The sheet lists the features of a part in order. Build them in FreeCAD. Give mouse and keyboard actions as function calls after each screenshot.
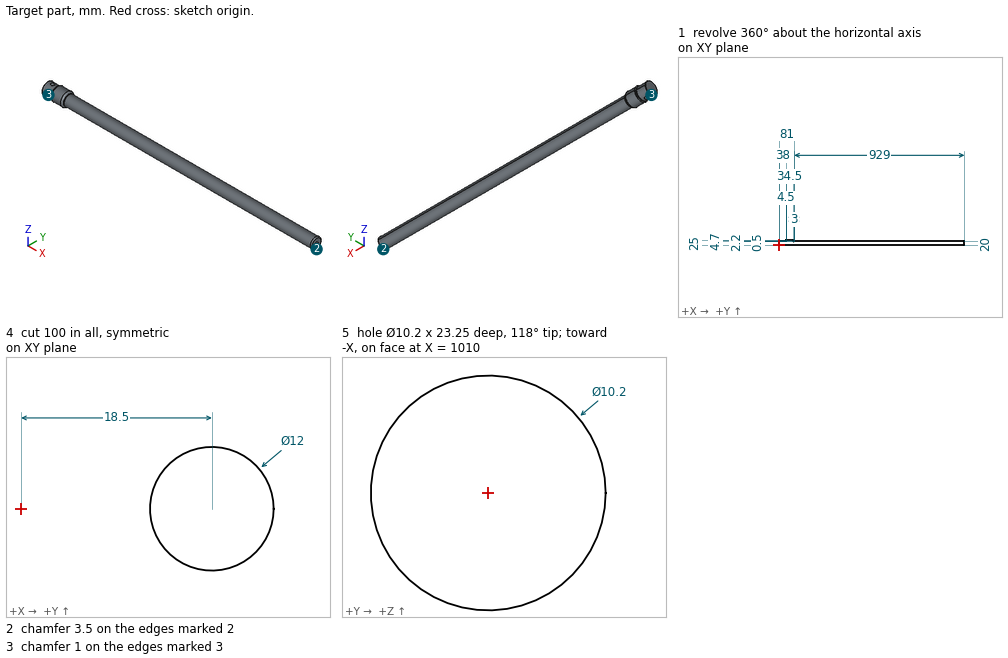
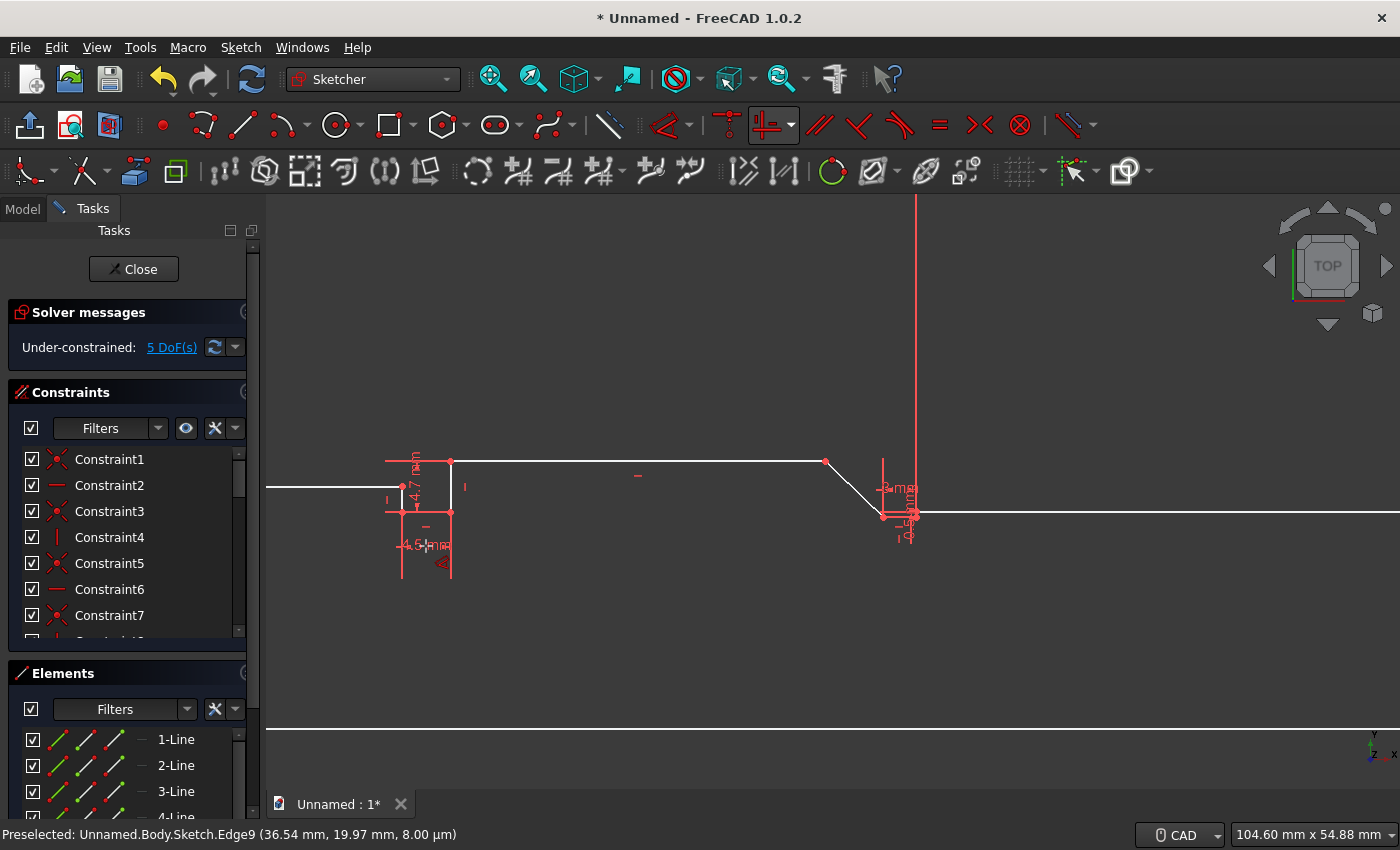
scroll(402, 502, up, 3)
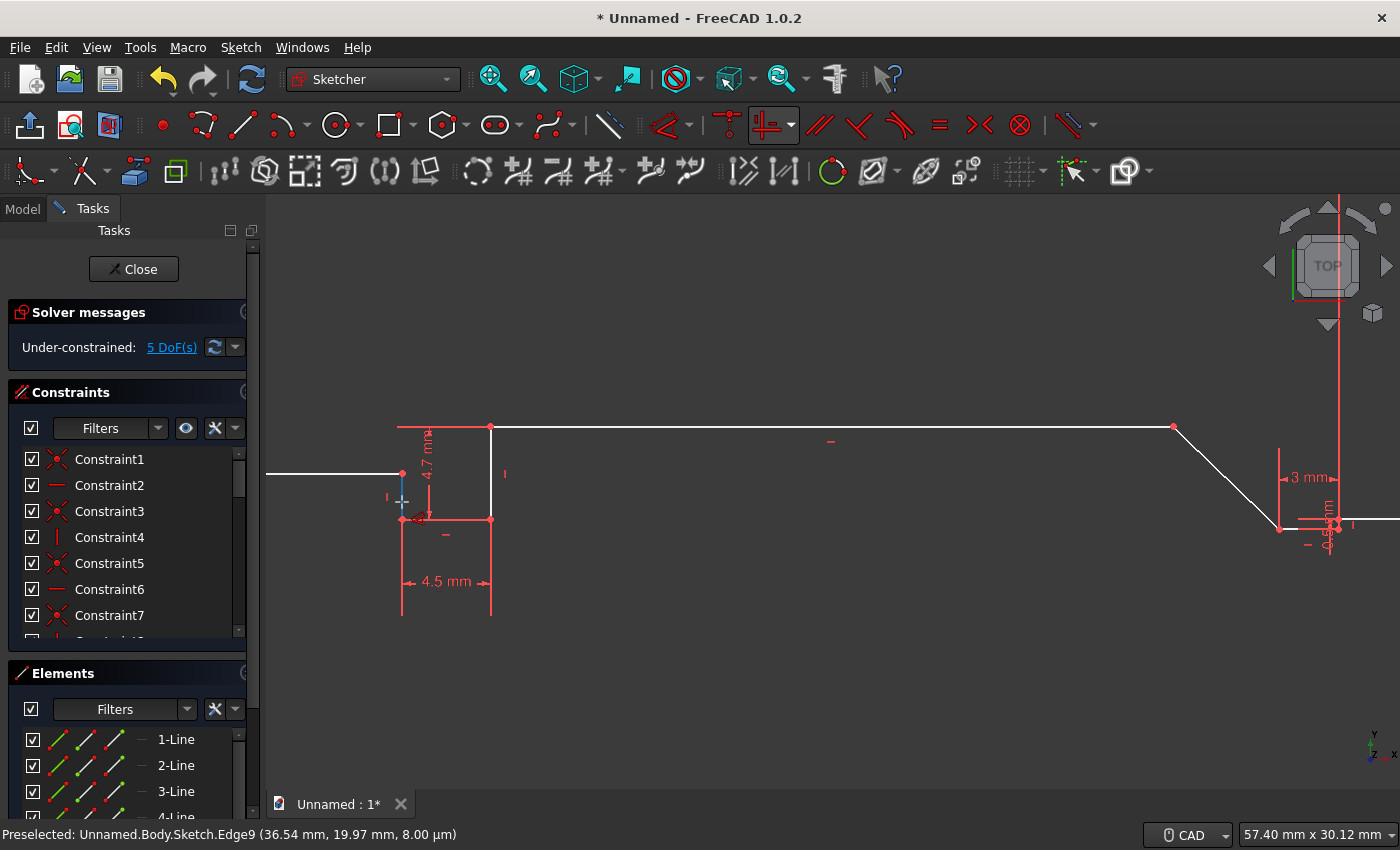
click(402, 501)
click(368, 497)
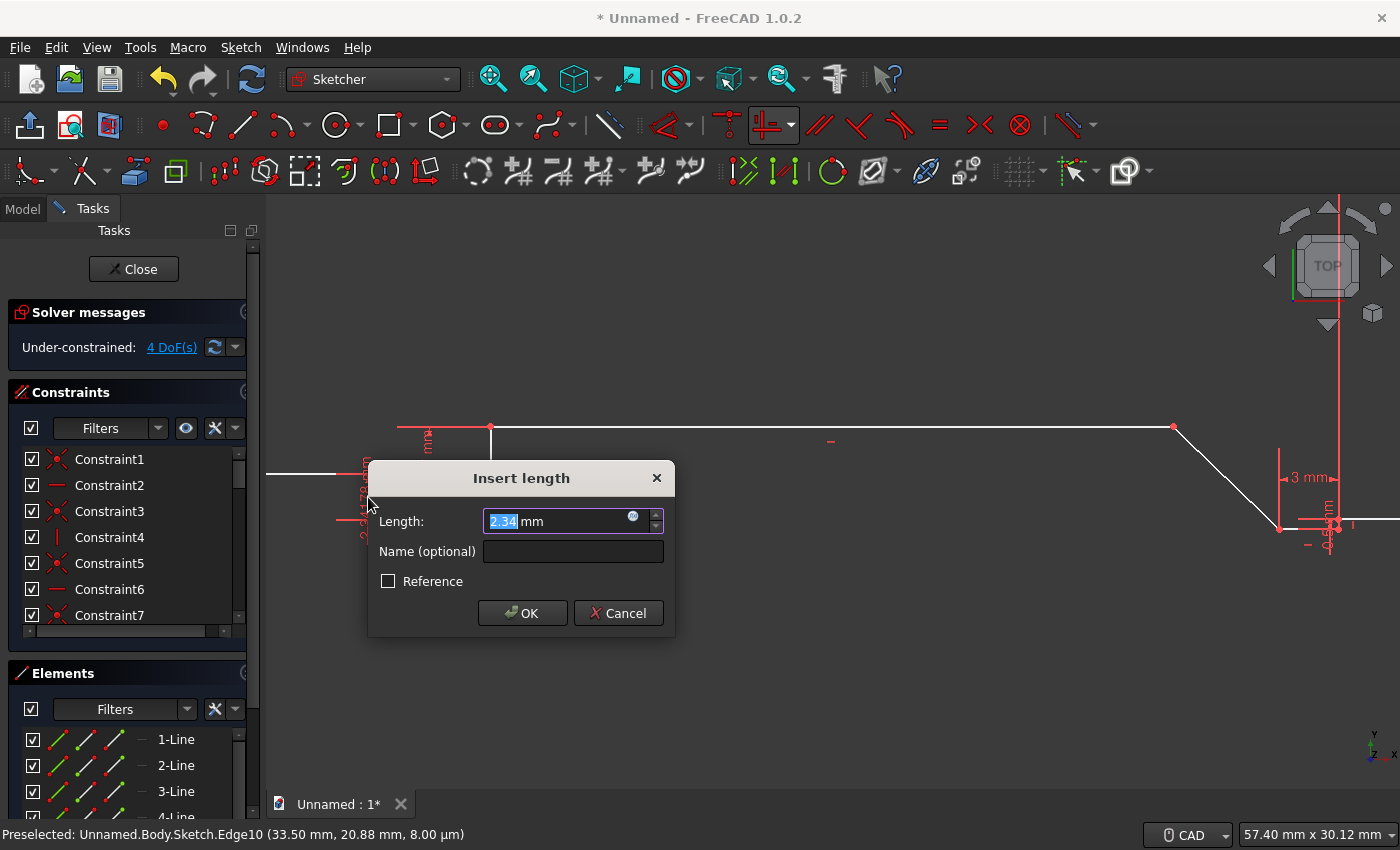
text(2.2)
key(Return)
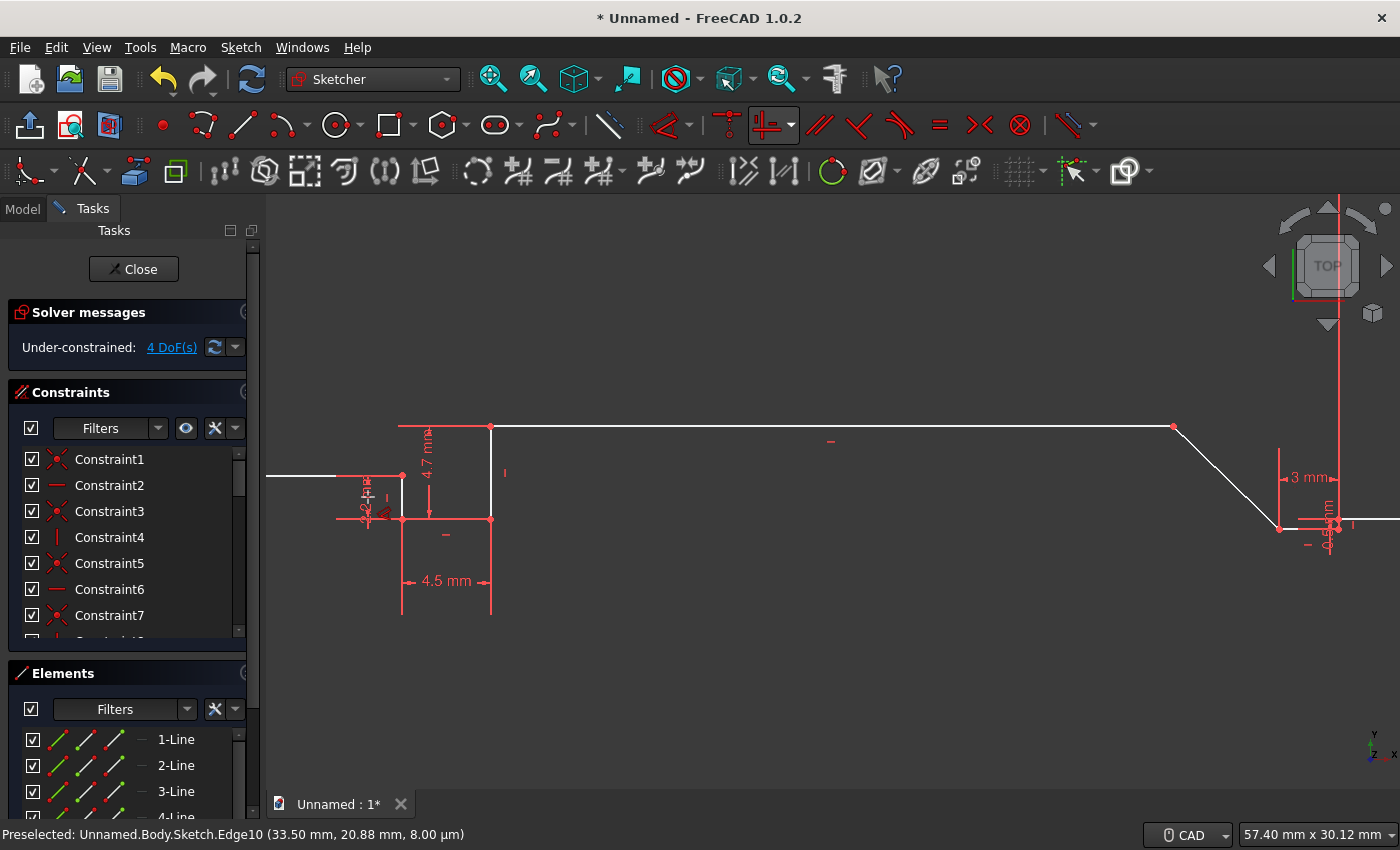
scroll(384, 484, down, 16)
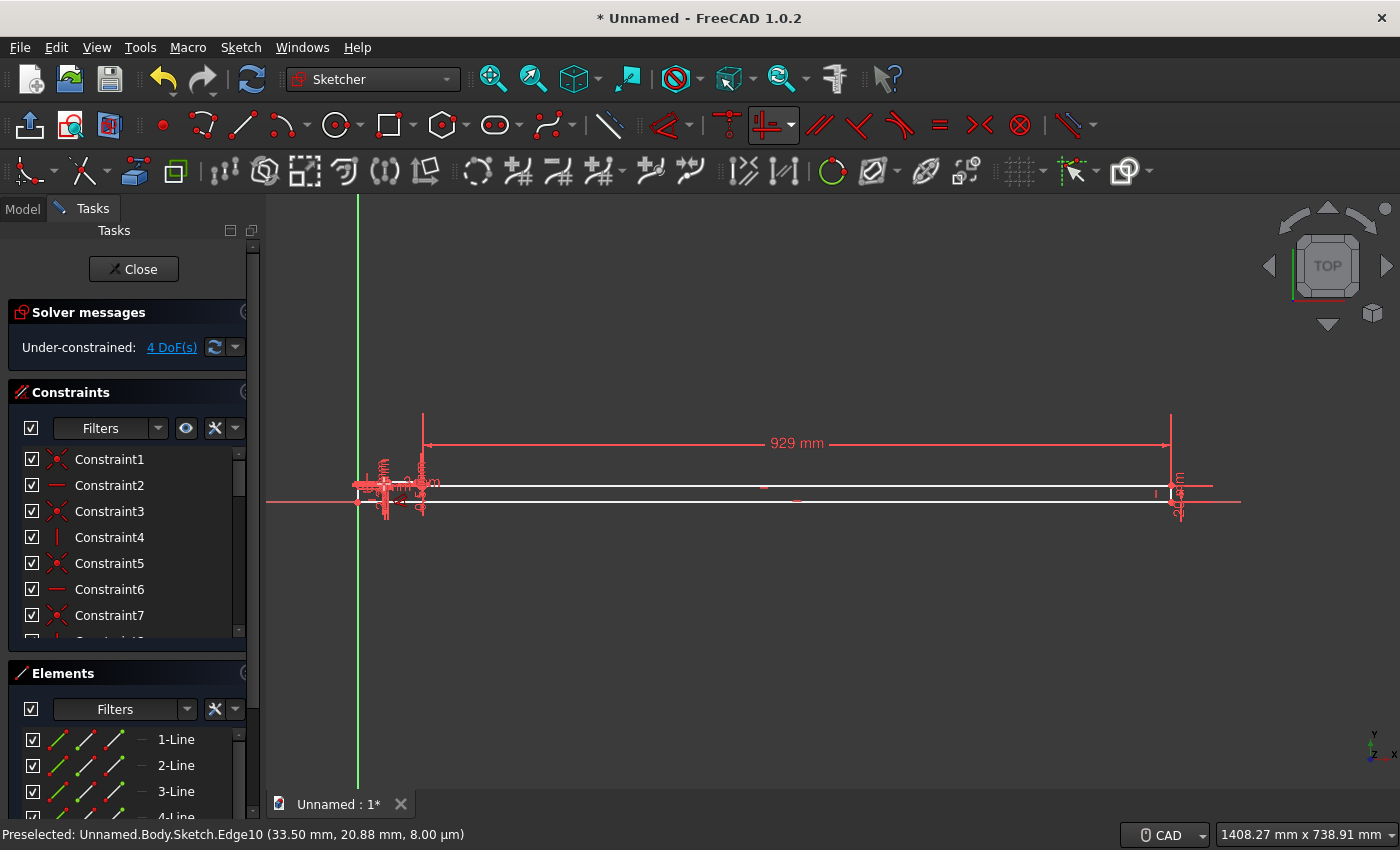
scroll(423, 486, up, 13)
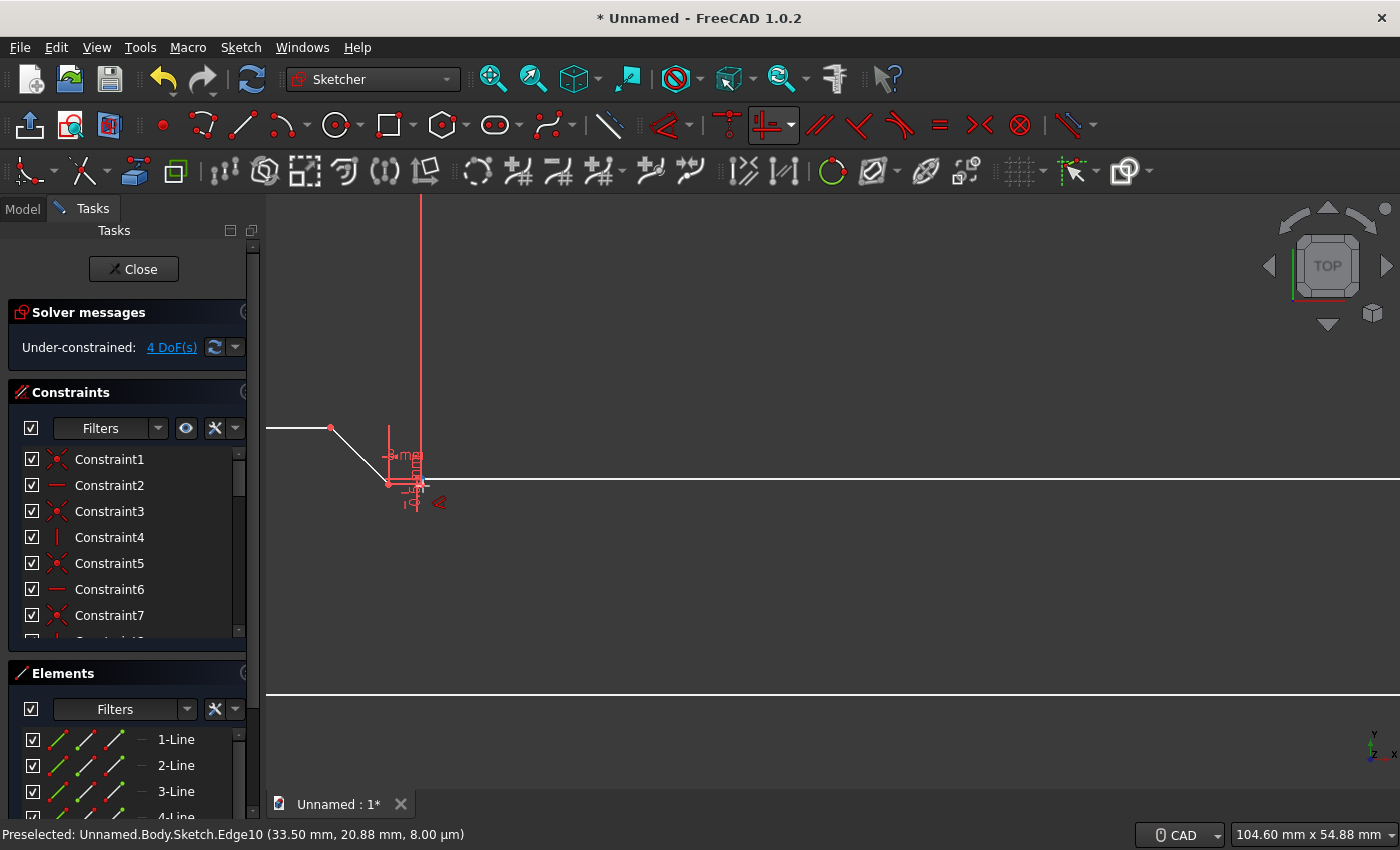
click(421, 479)
click(358, 729)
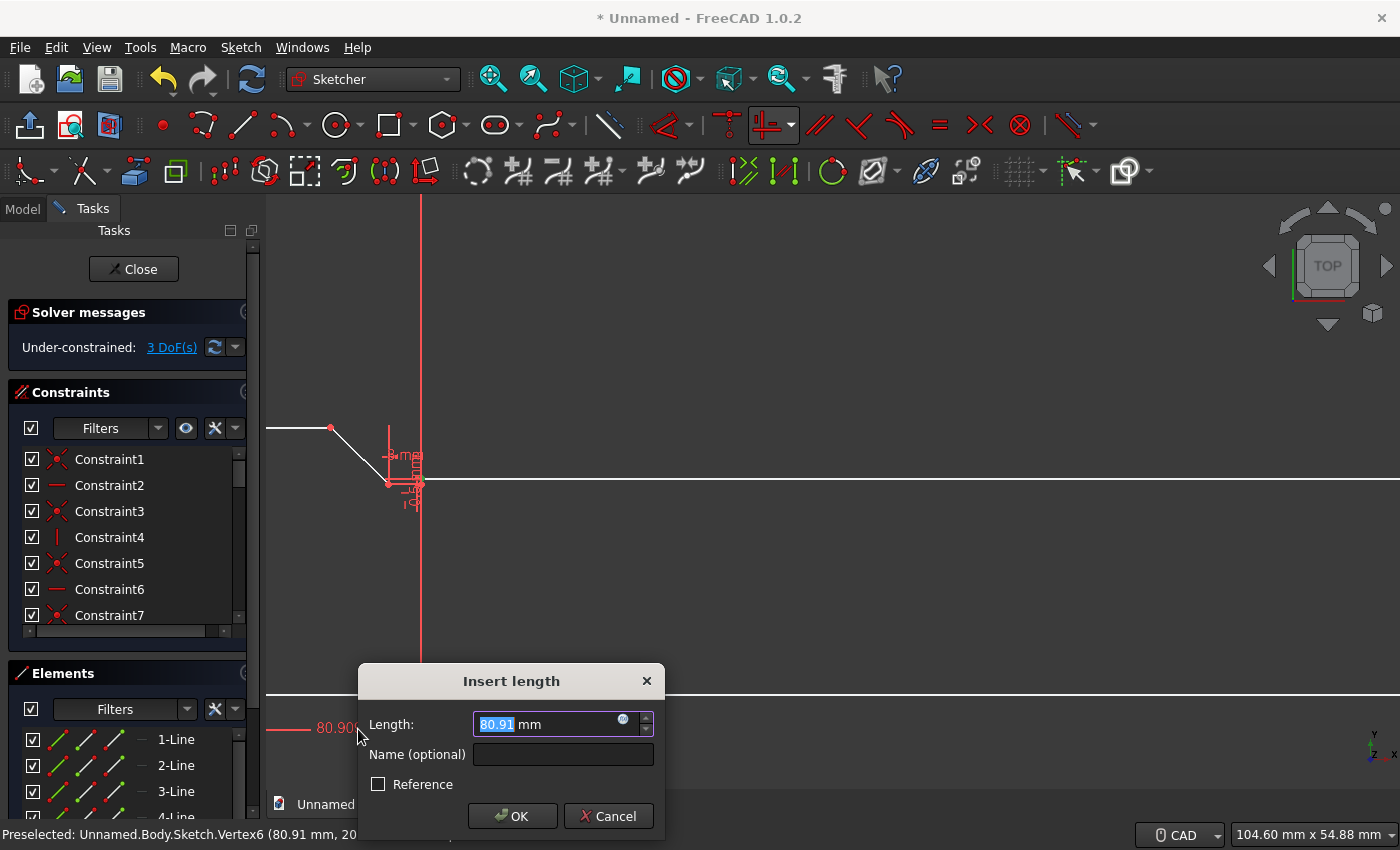
text(81)
key(Return)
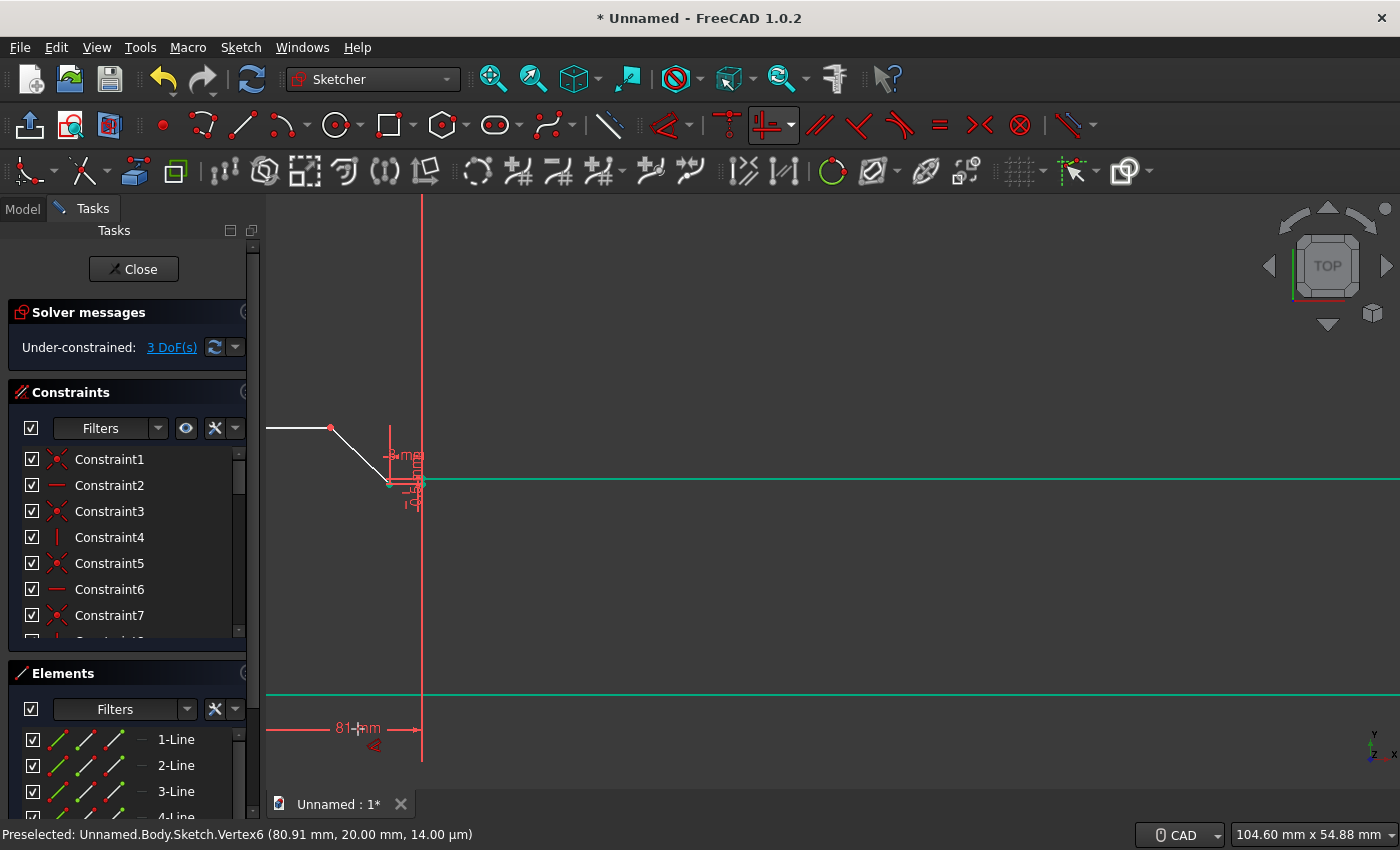
scroll(489, 487, down, 14)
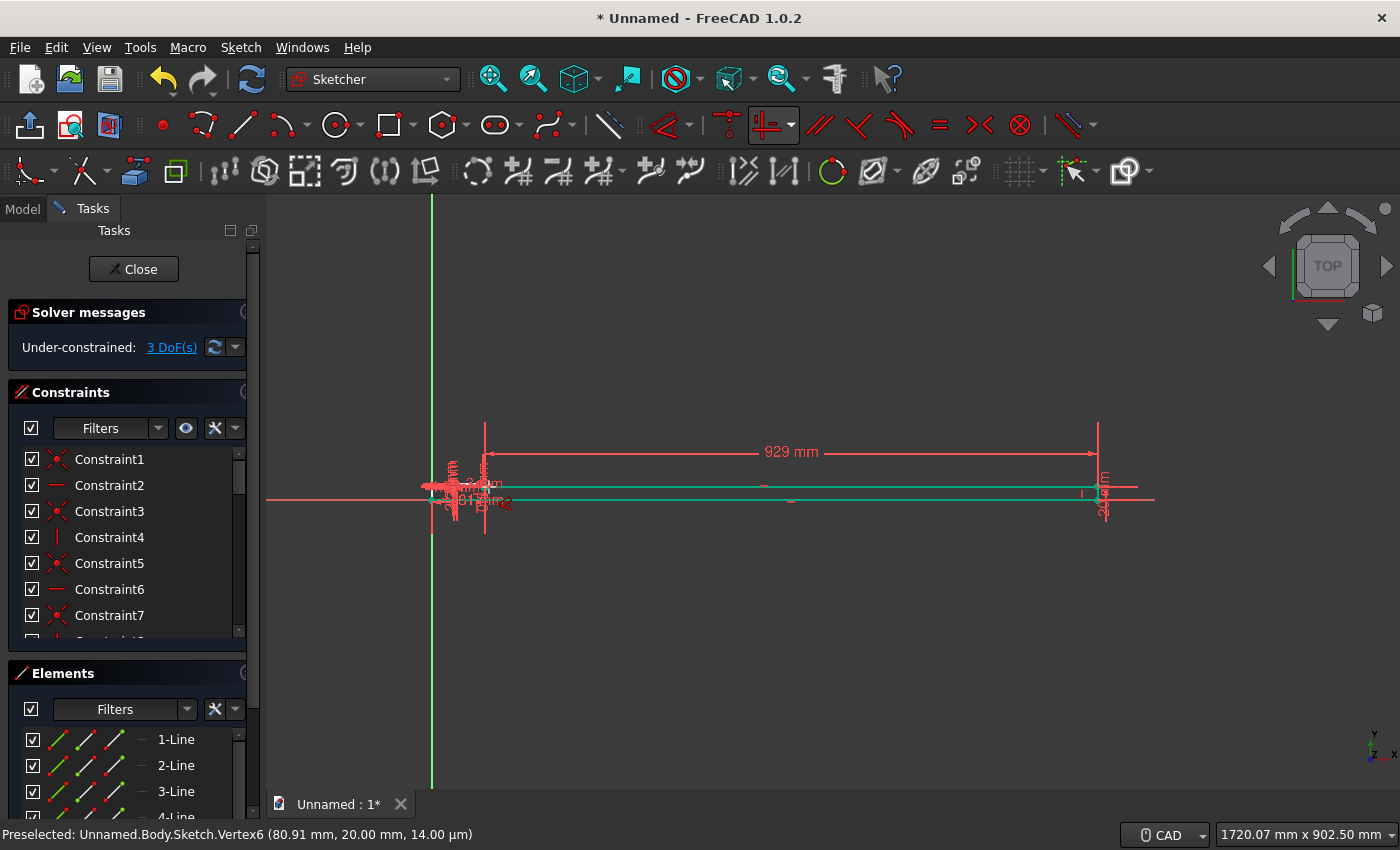
scroll(480, 484, up, 5)